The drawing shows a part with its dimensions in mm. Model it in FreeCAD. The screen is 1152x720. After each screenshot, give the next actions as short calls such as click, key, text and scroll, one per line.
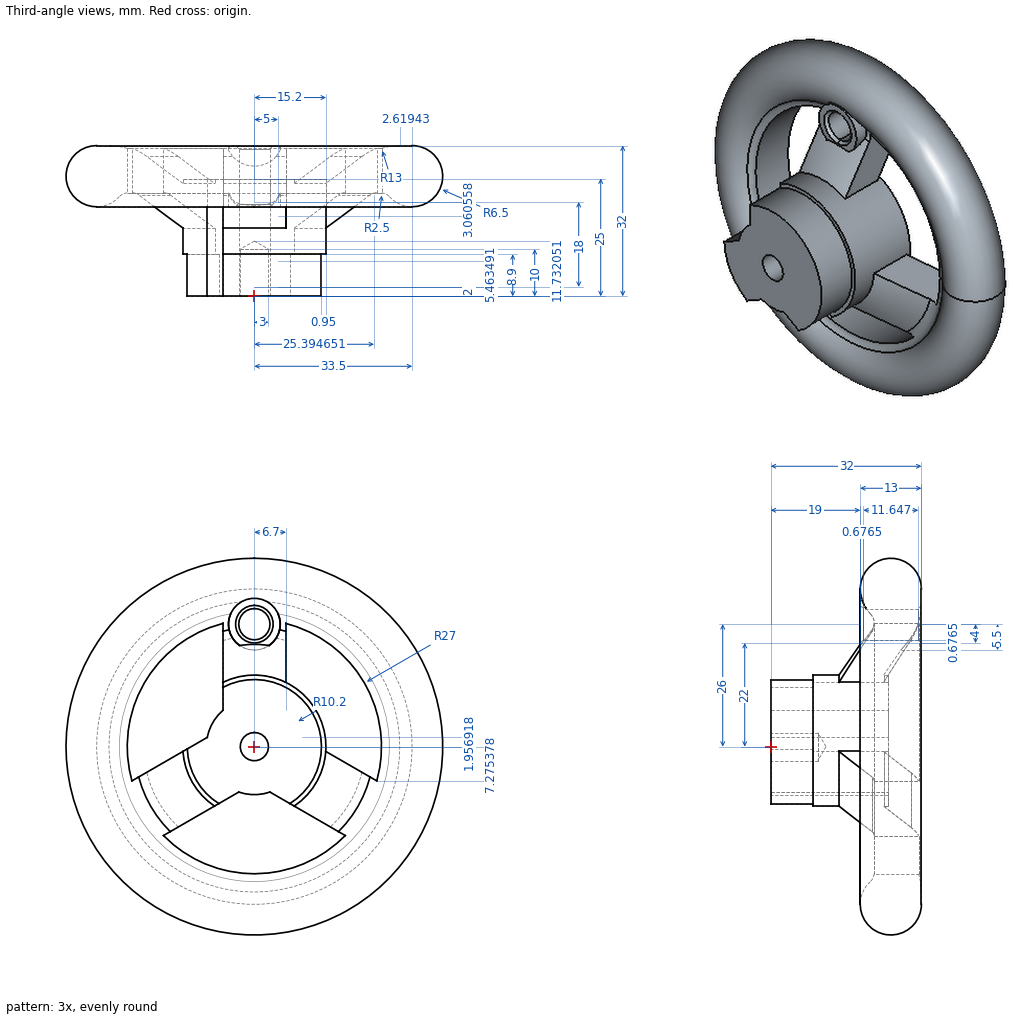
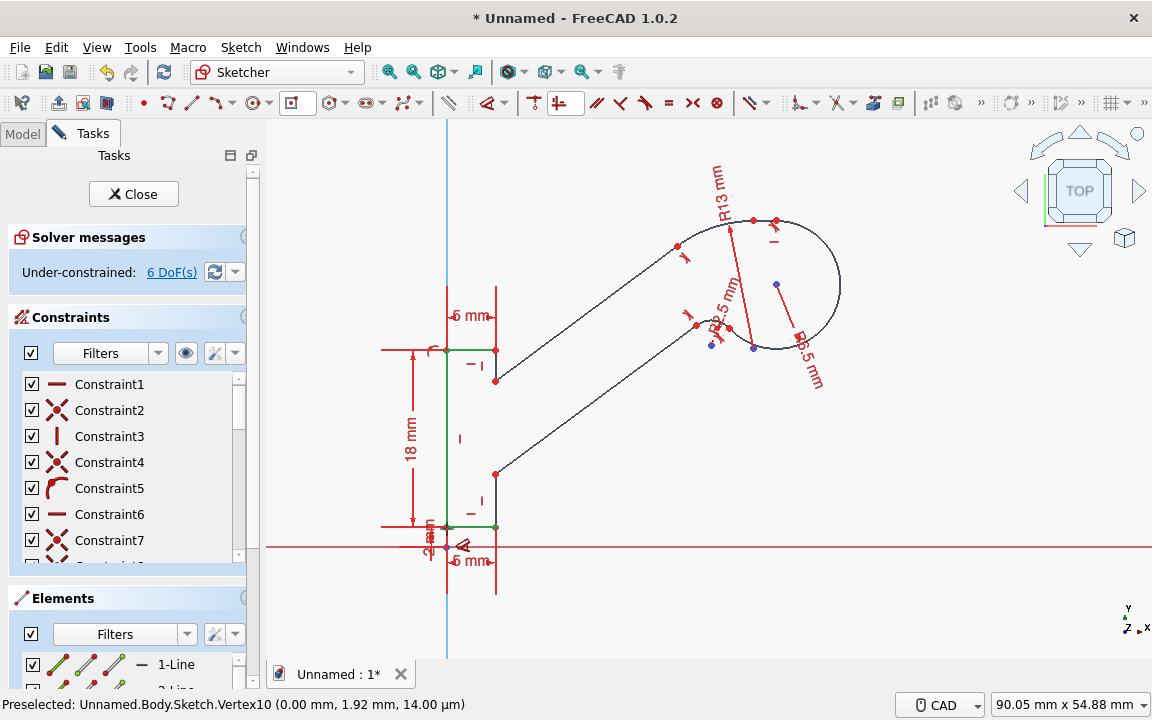
click(776, 221)
click(413, 384)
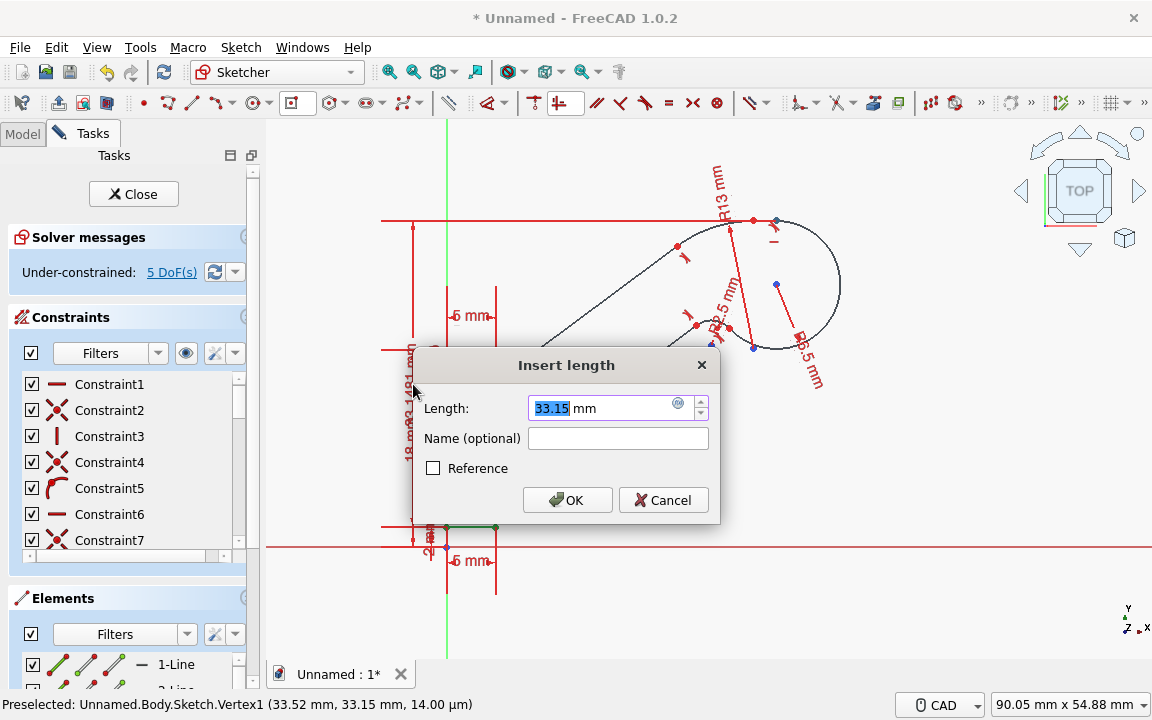
text(32)
key(Return)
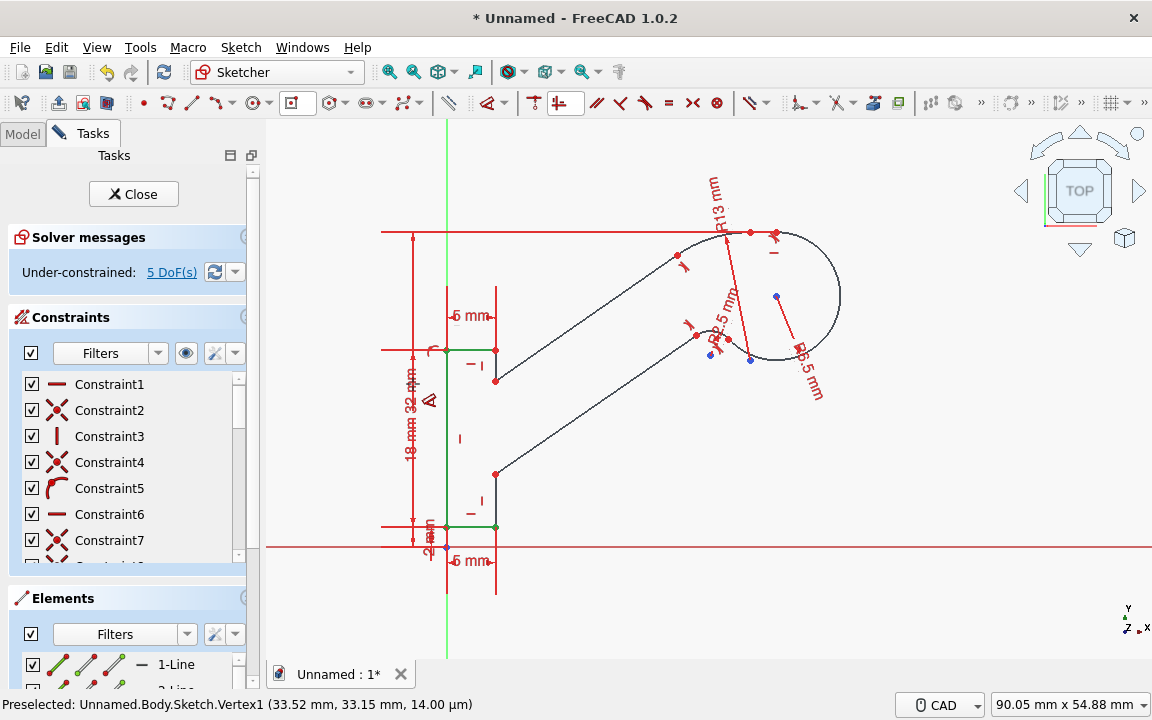
click(776, 232)
click(611, 581)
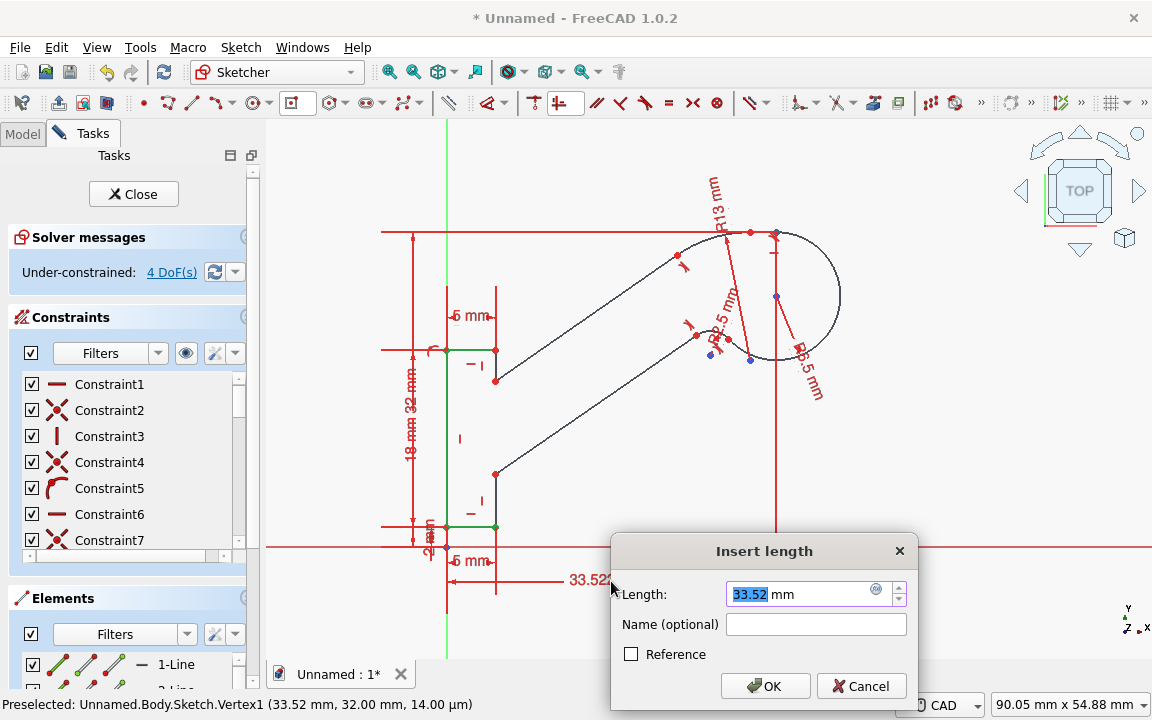
text(33.5)
key(Return)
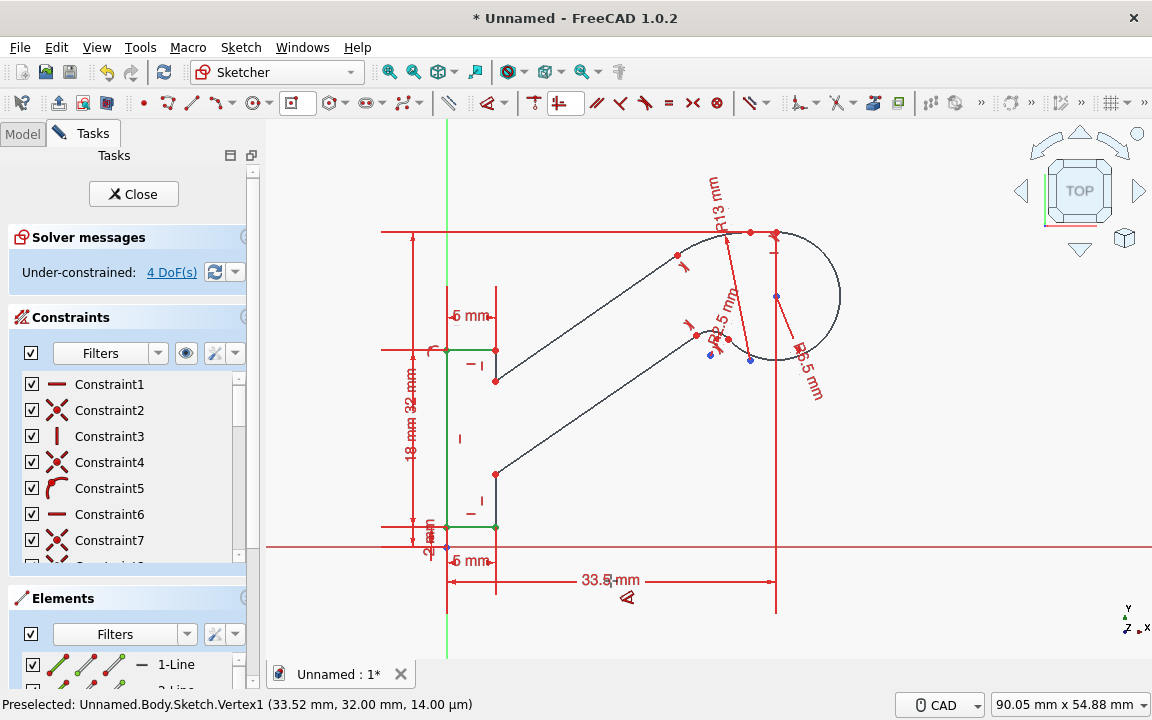
scroll(766, 232, up, 3)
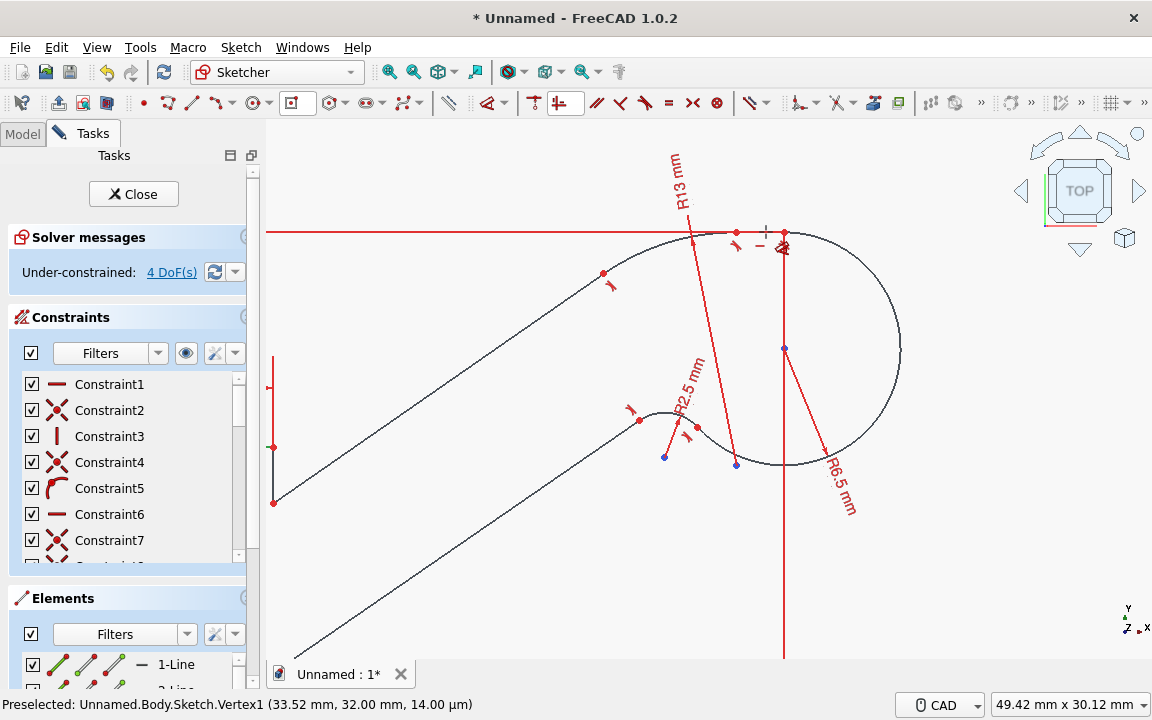
click(765, 232)
click(760, 198)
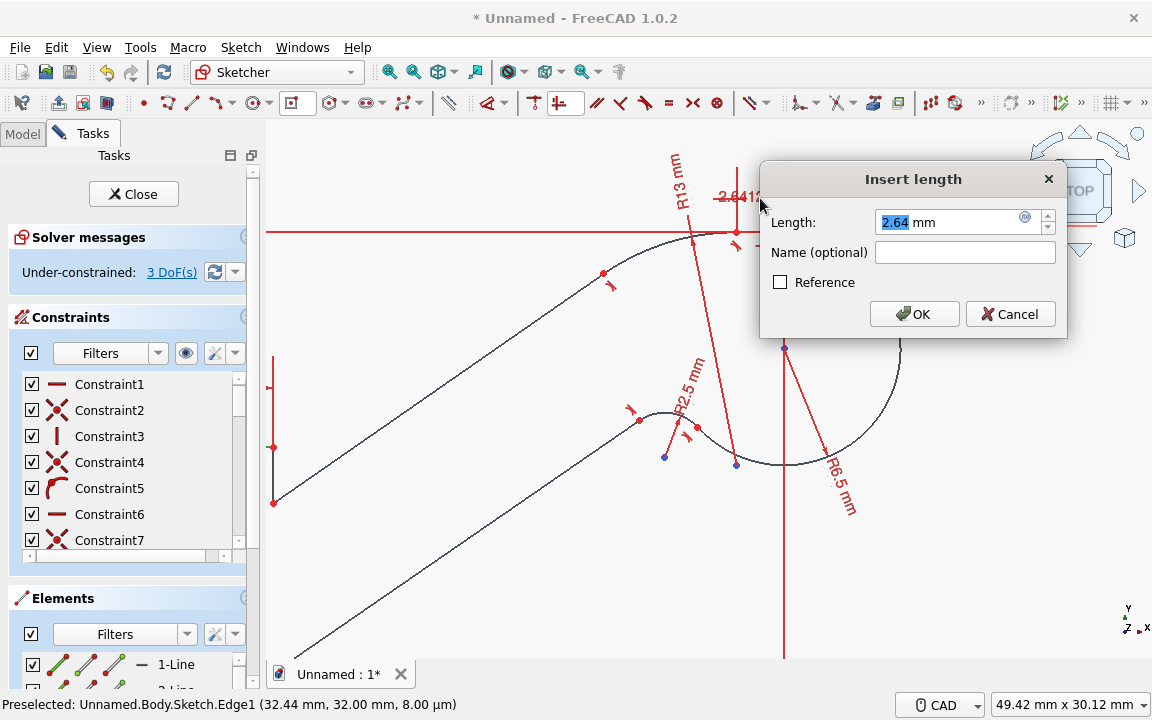
text(2.61943)
key(Return)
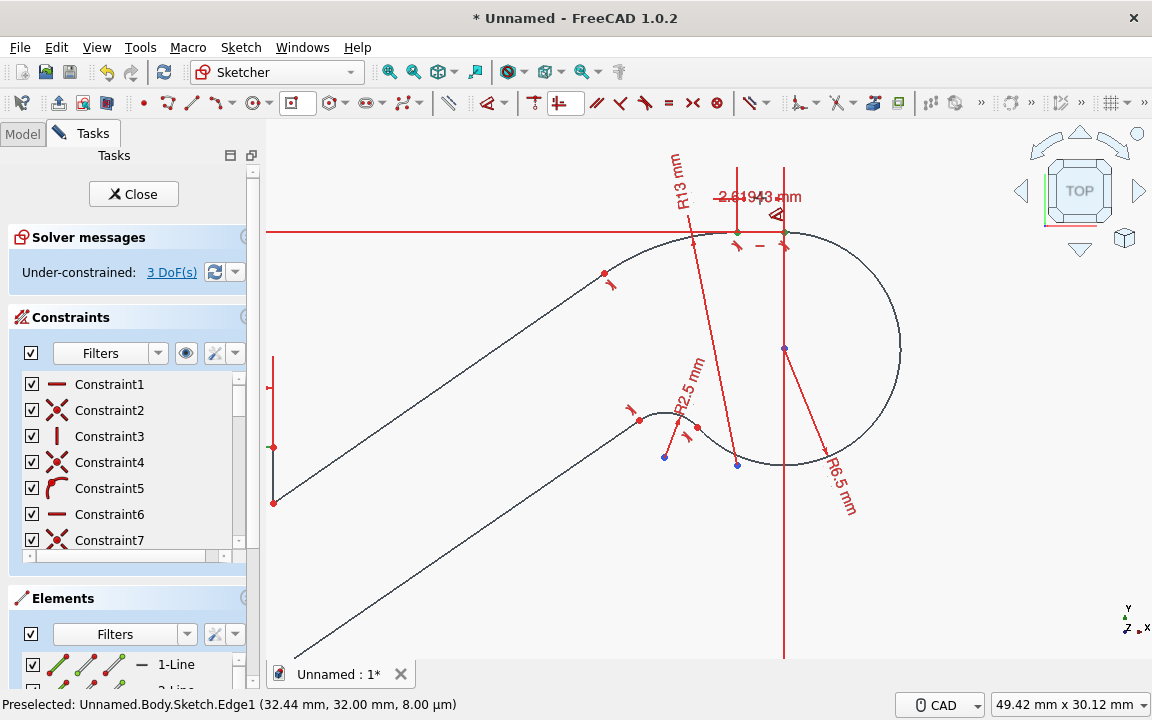
scroll(766, 231, down, 3)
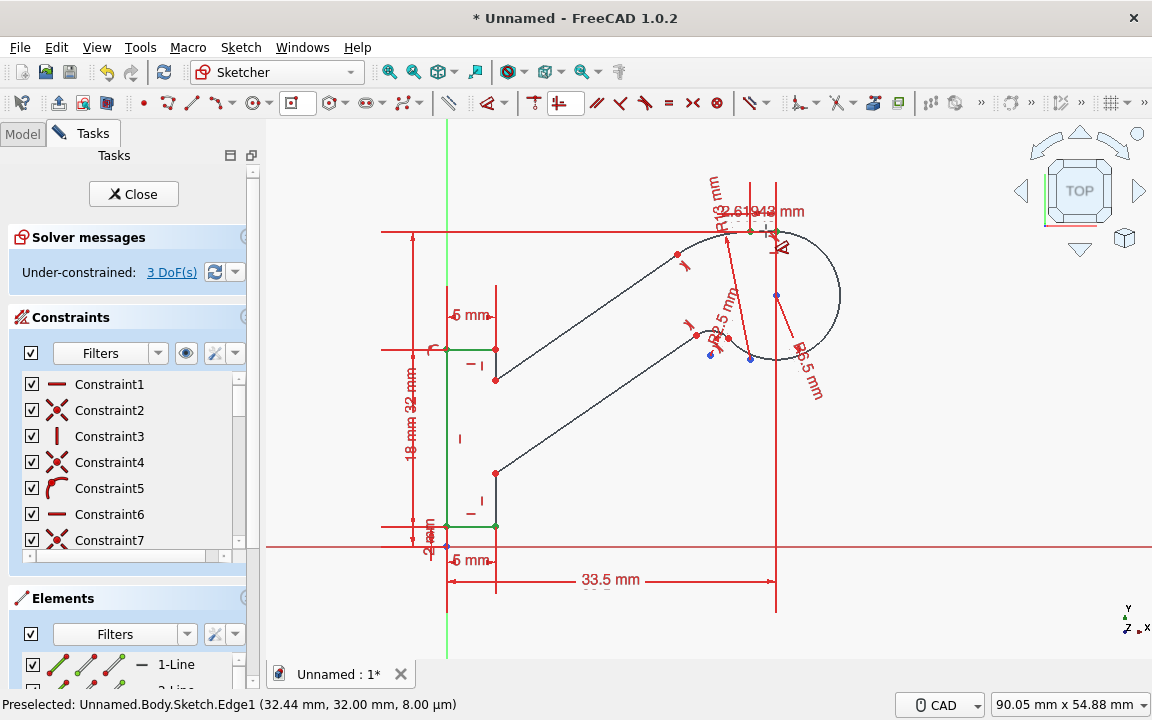
scroll(496, 371, up, 3)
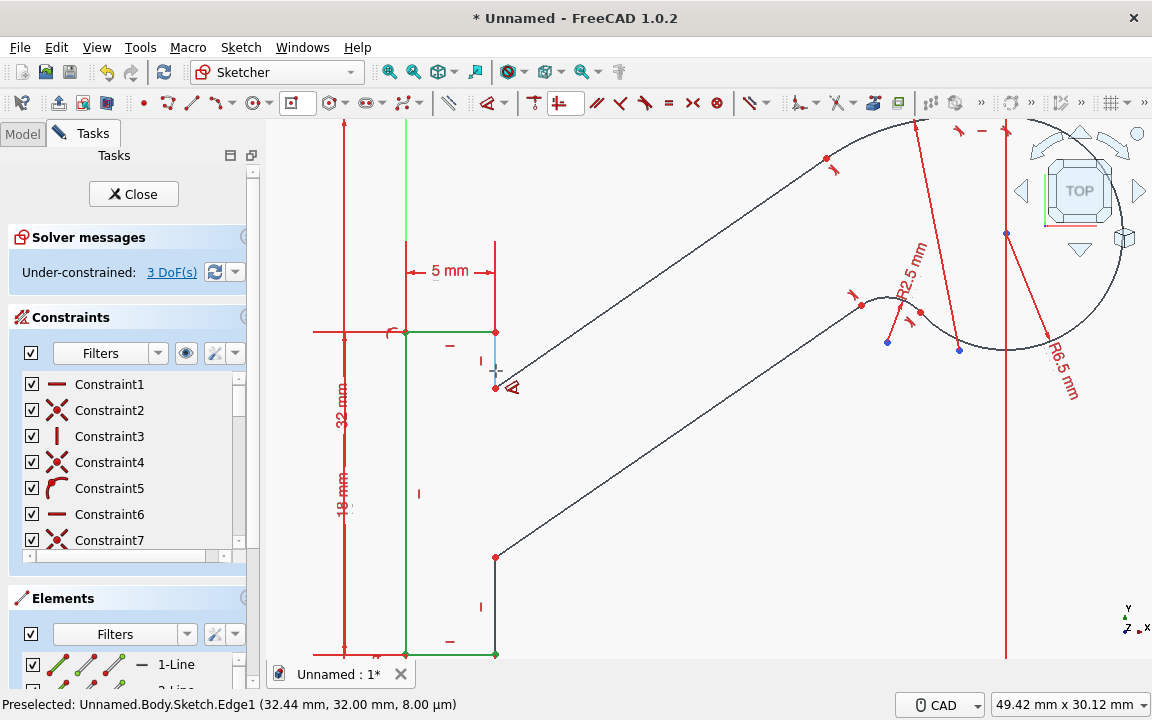
click(495, 372)
click(461, 360)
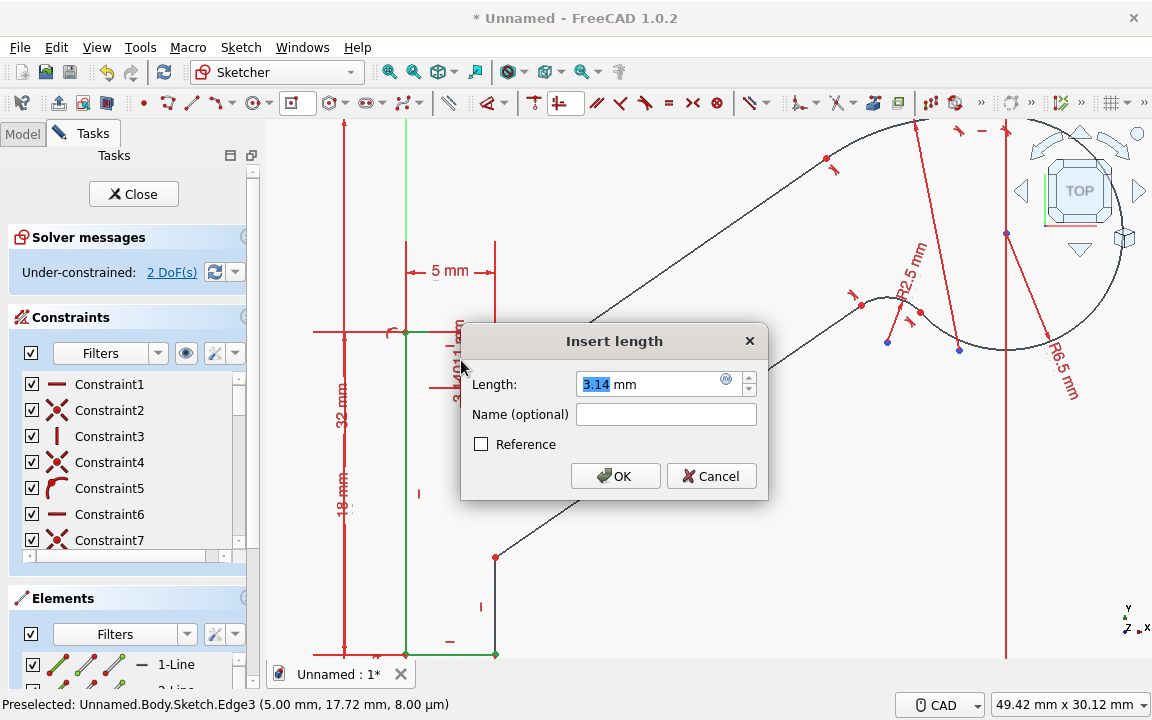
text(3.060558)
key(Return)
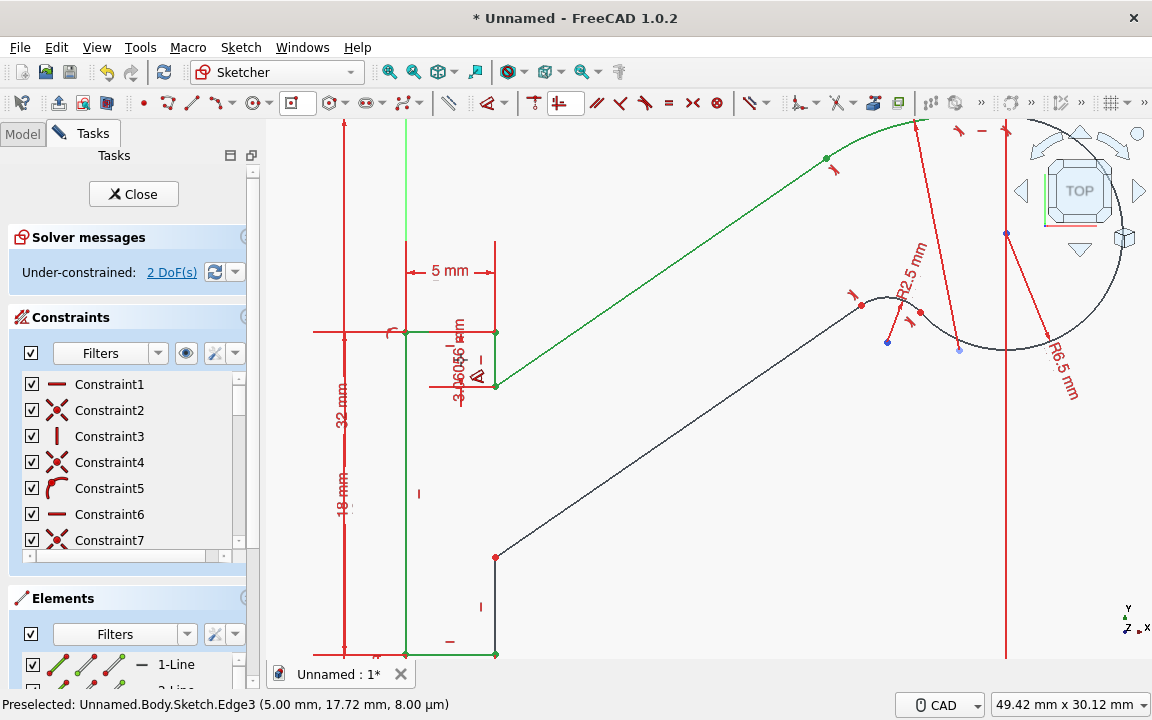
click(495, 626)
click(461, 594)